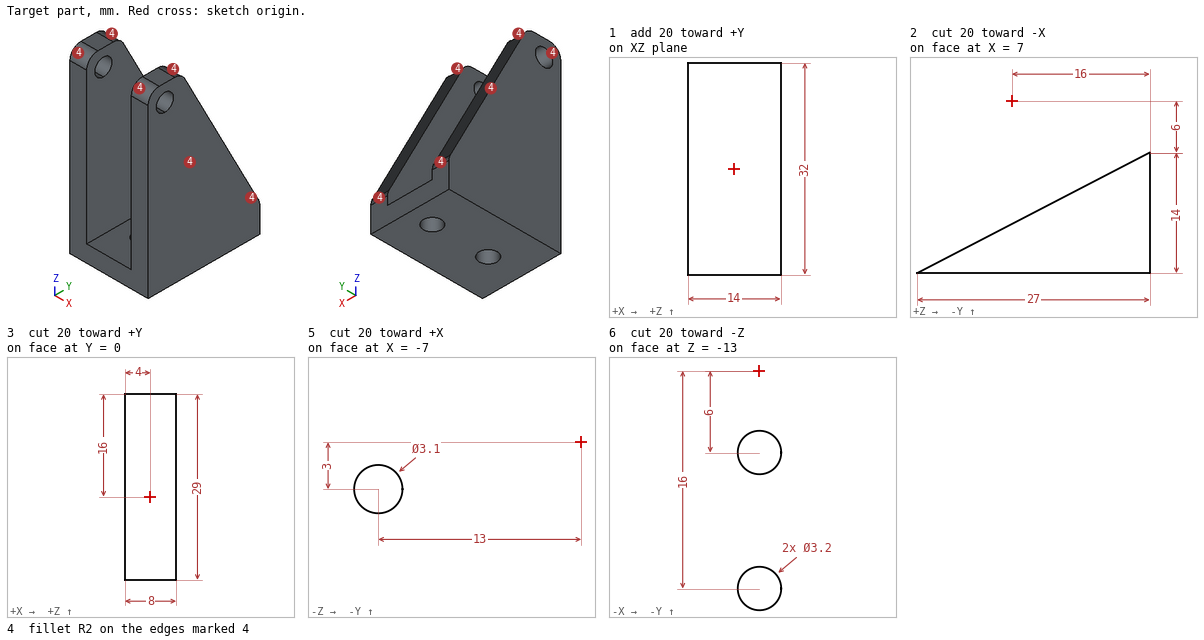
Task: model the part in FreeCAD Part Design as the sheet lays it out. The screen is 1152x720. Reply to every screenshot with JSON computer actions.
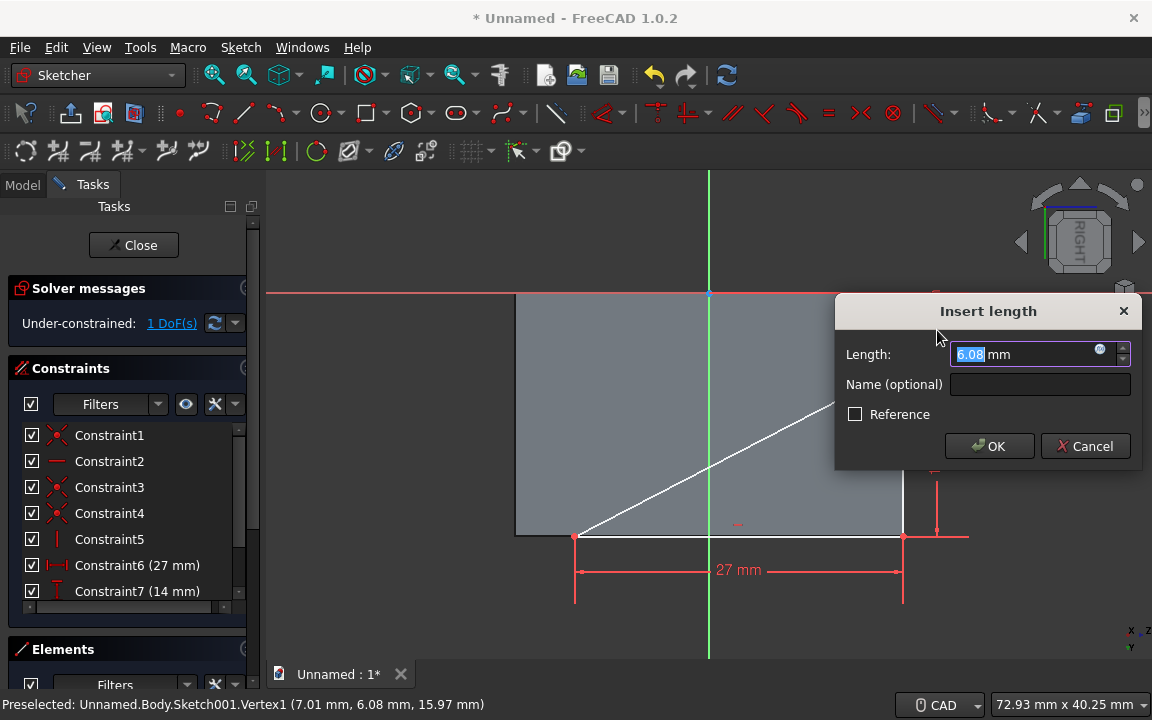
{"action": "type", "text": "6"}
{"action": "key", "text": "Return"}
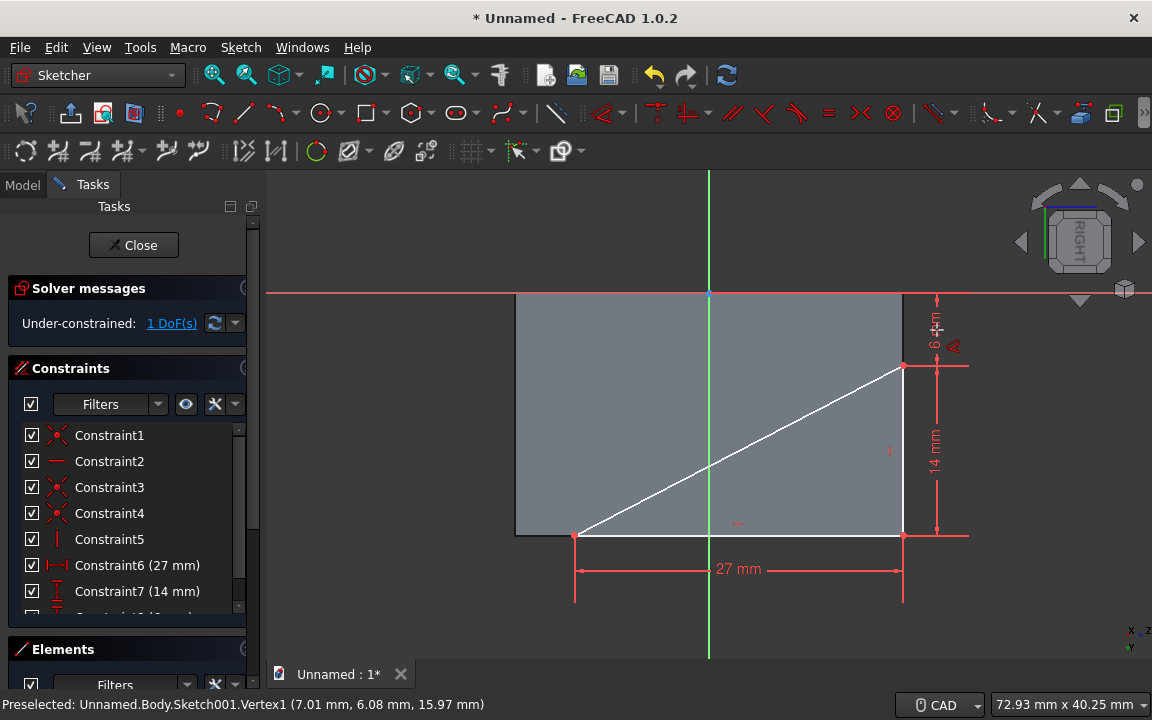
{"action": "left_click", "coordinate": [903, 366]}
{"action": "left_click", "coordinate": [806, 259]}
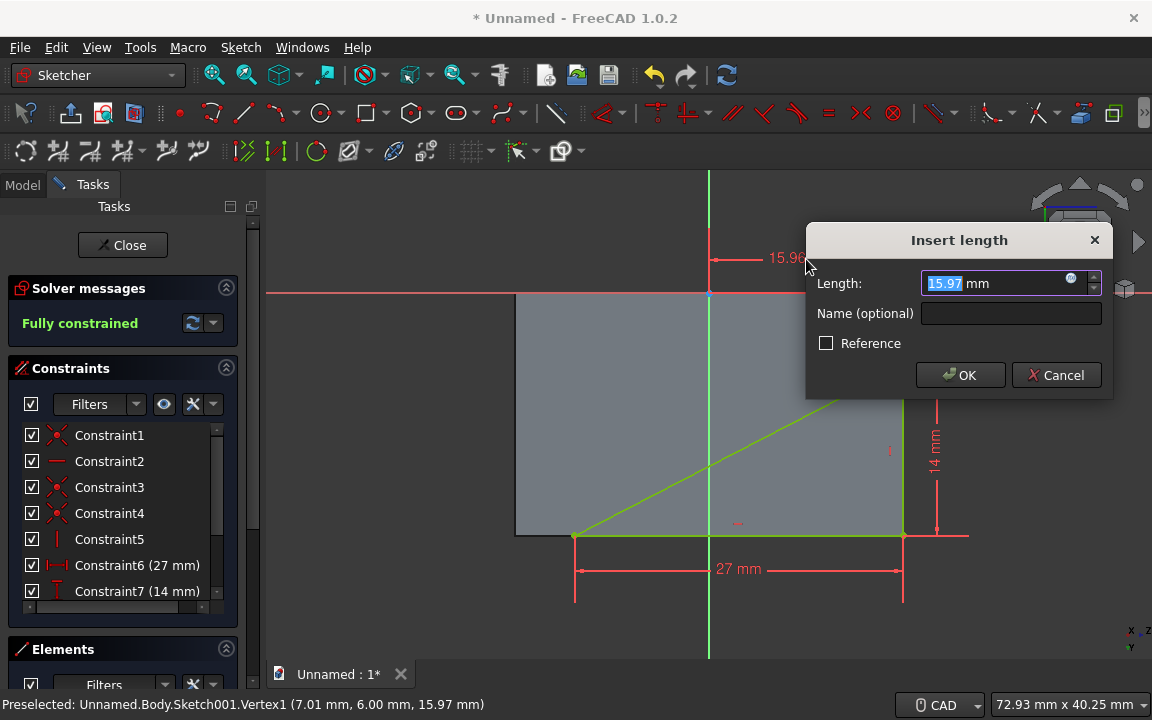
{"action": "type", "text": "16"}
{"action": "key", "text": "Return"}
{"action": "key", "text": "Escape"}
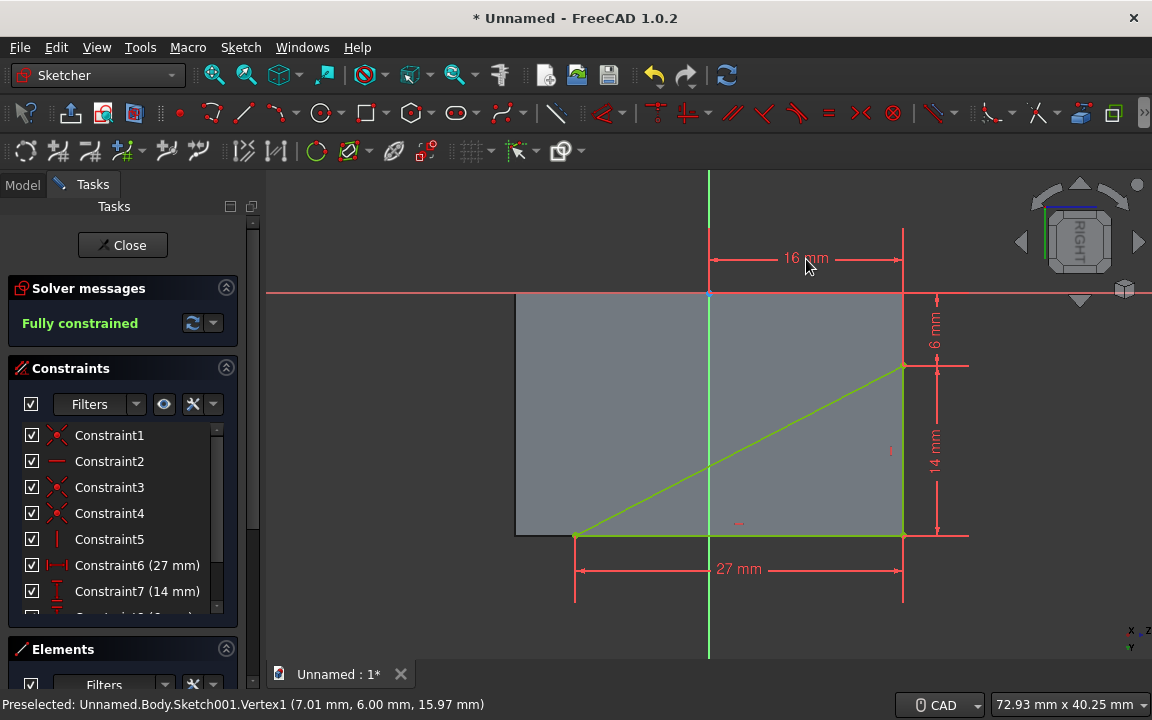
{"action": "left_click", "coordinate": [123, 245]}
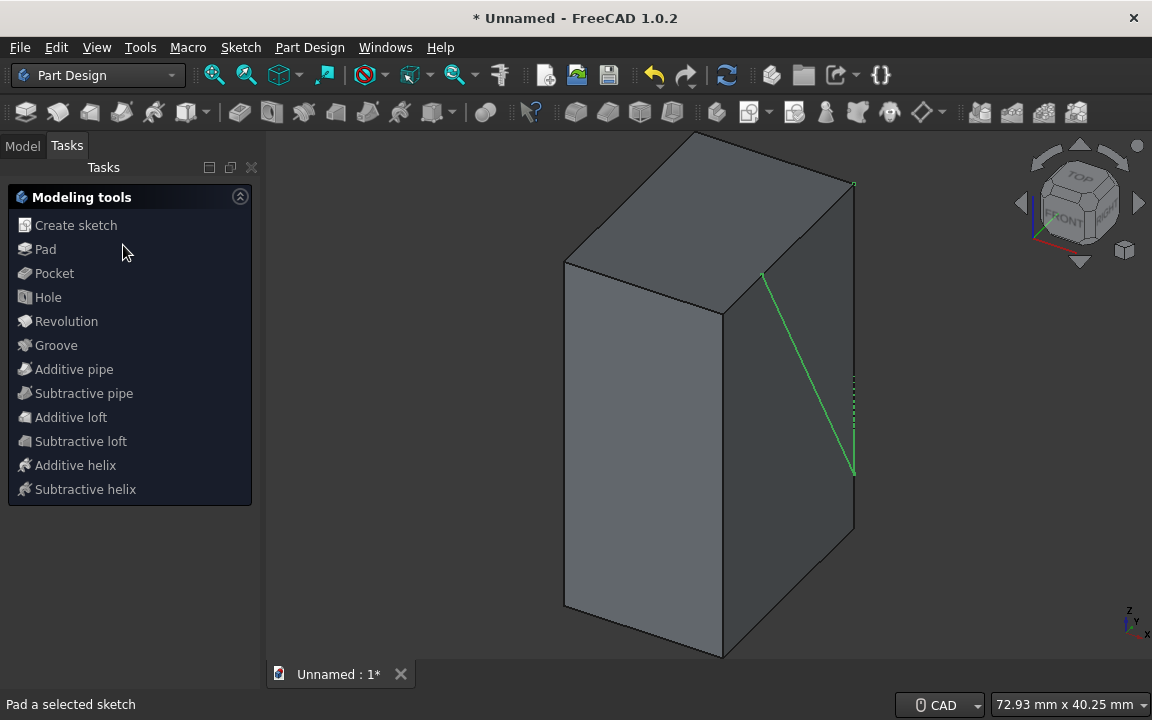
{"action": "left_click", "coordinate": [240, 112]}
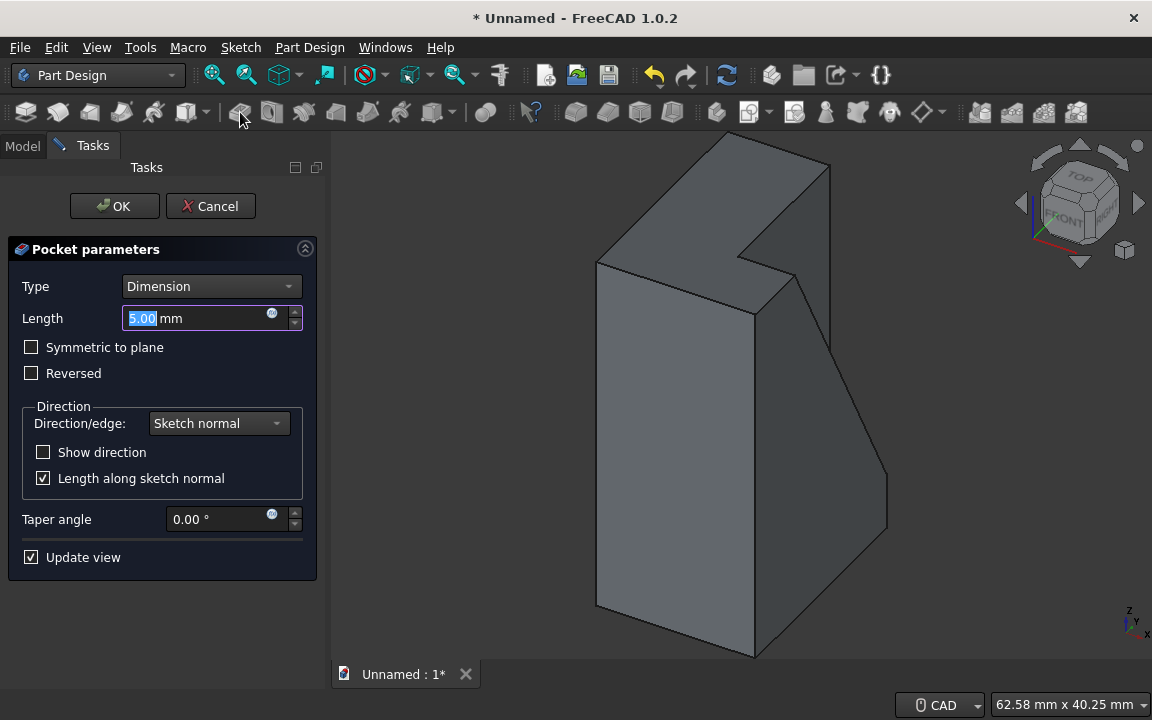
{"action": "type", "text": "20"}
{"action": "key", "text": "Tab"}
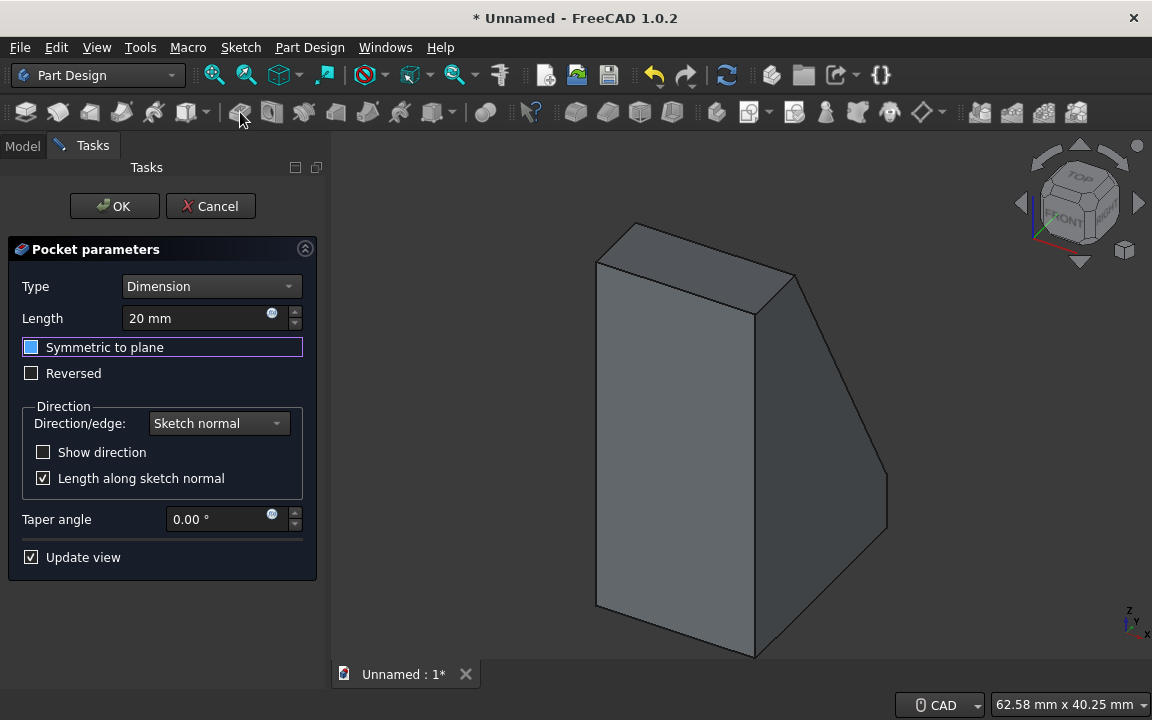
{"action": "left_click", "coordinate": [115, 206]}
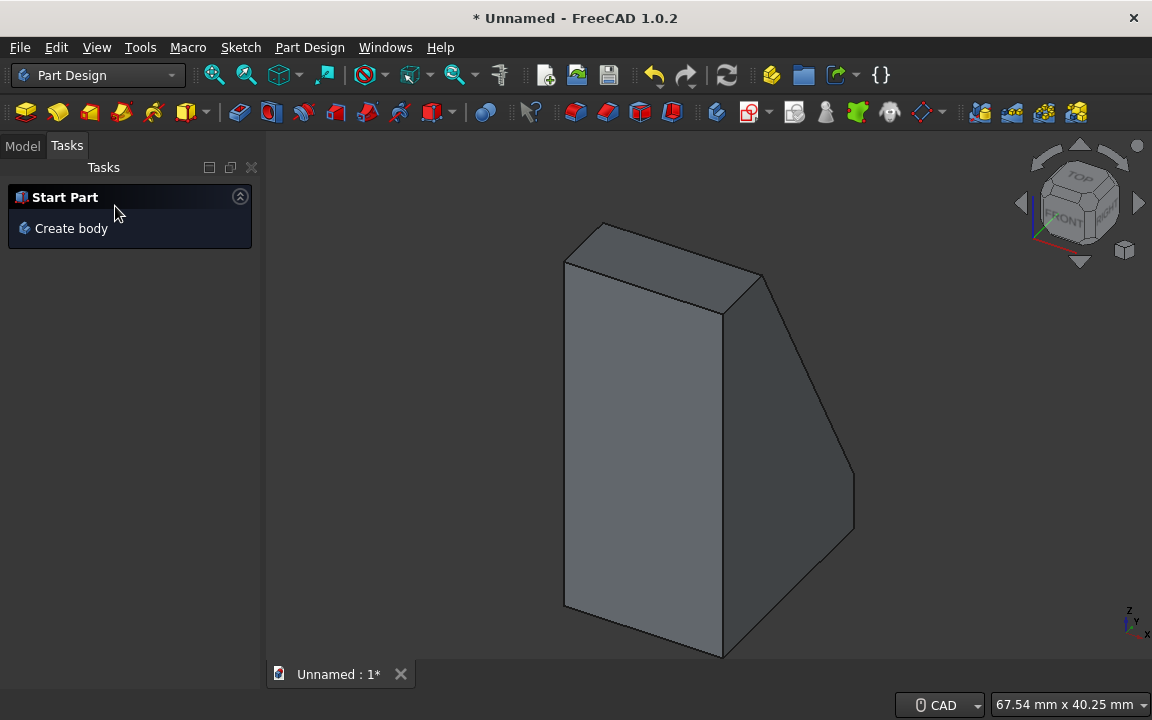
{"action": "left_click", "coordinate": [643, 410]}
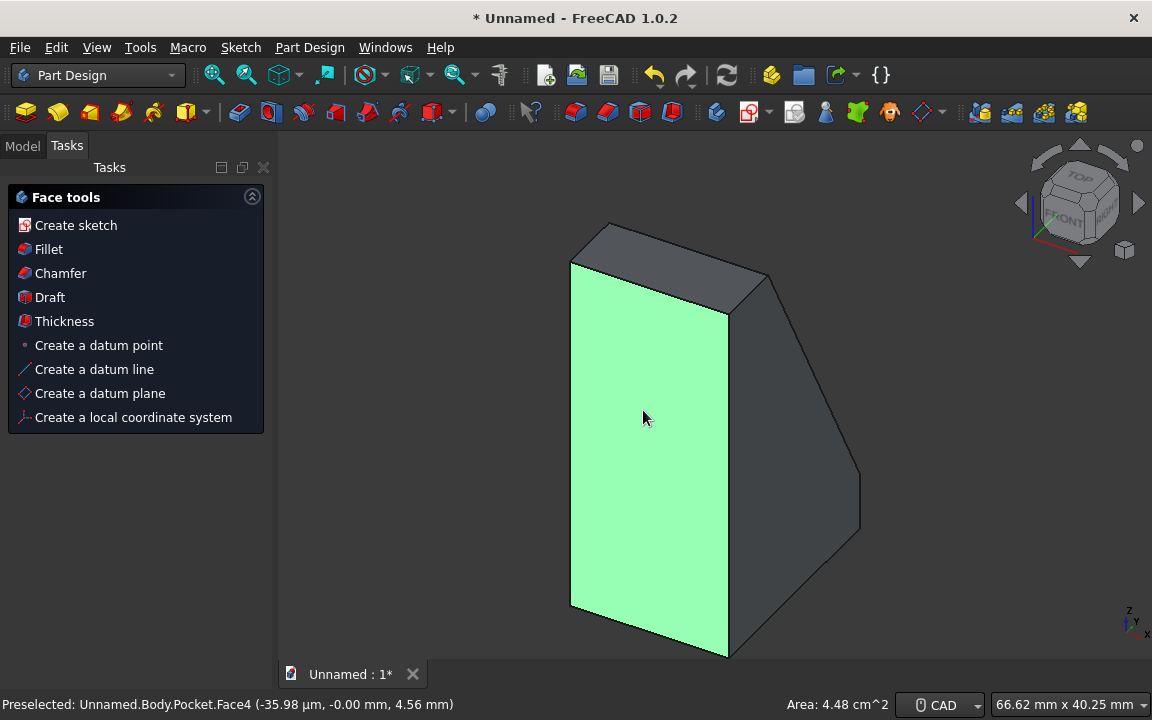
{"action": "left_click", "coordinate": [750, 112]}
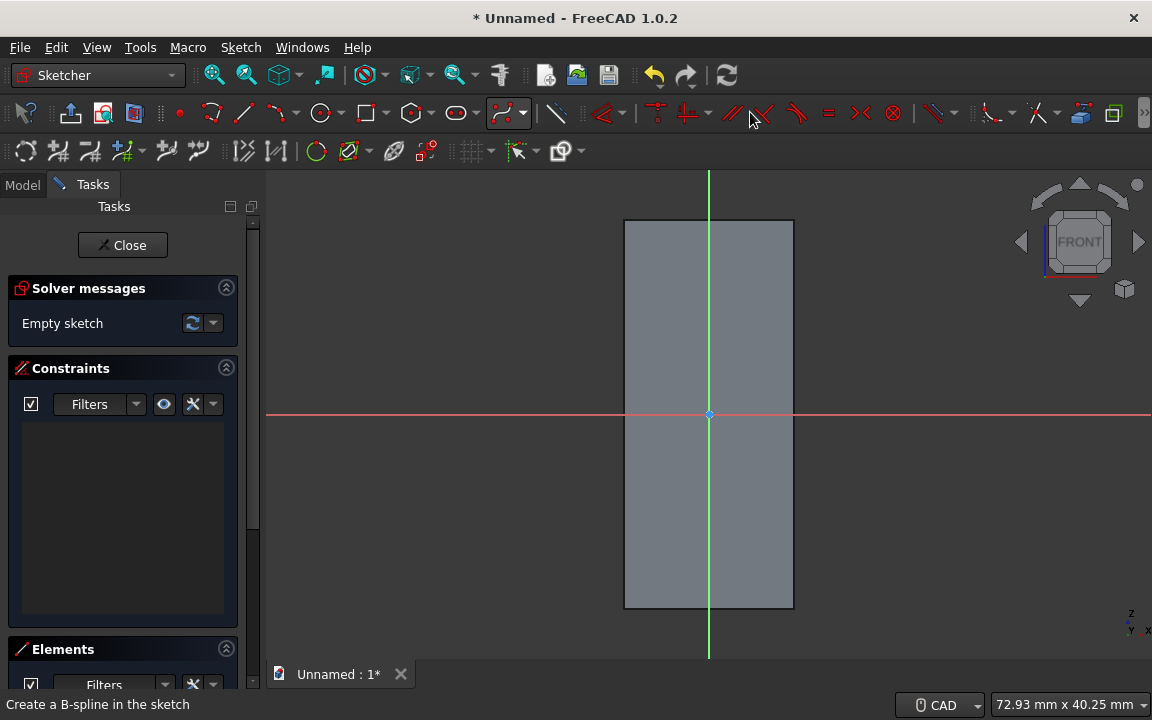
{"action": "scroll", "coordinate": [331, 497], "scroll_direction": "down", "scroll_amount": 1}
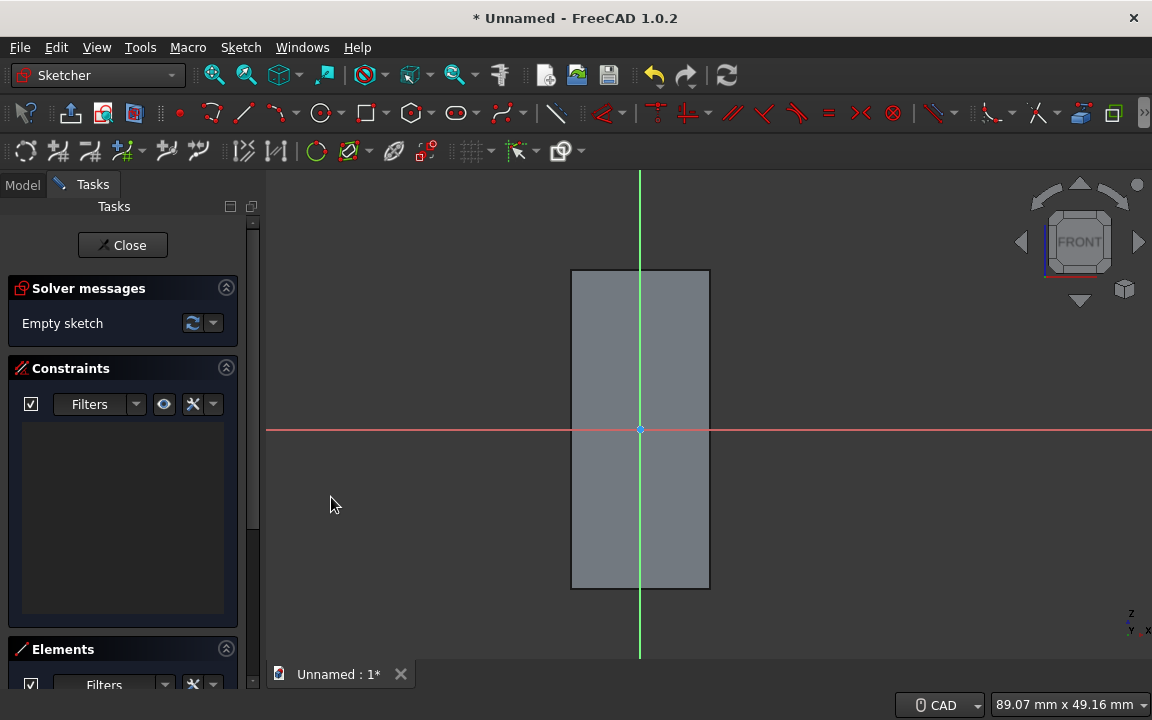
{"action": "key", "text": "g r"}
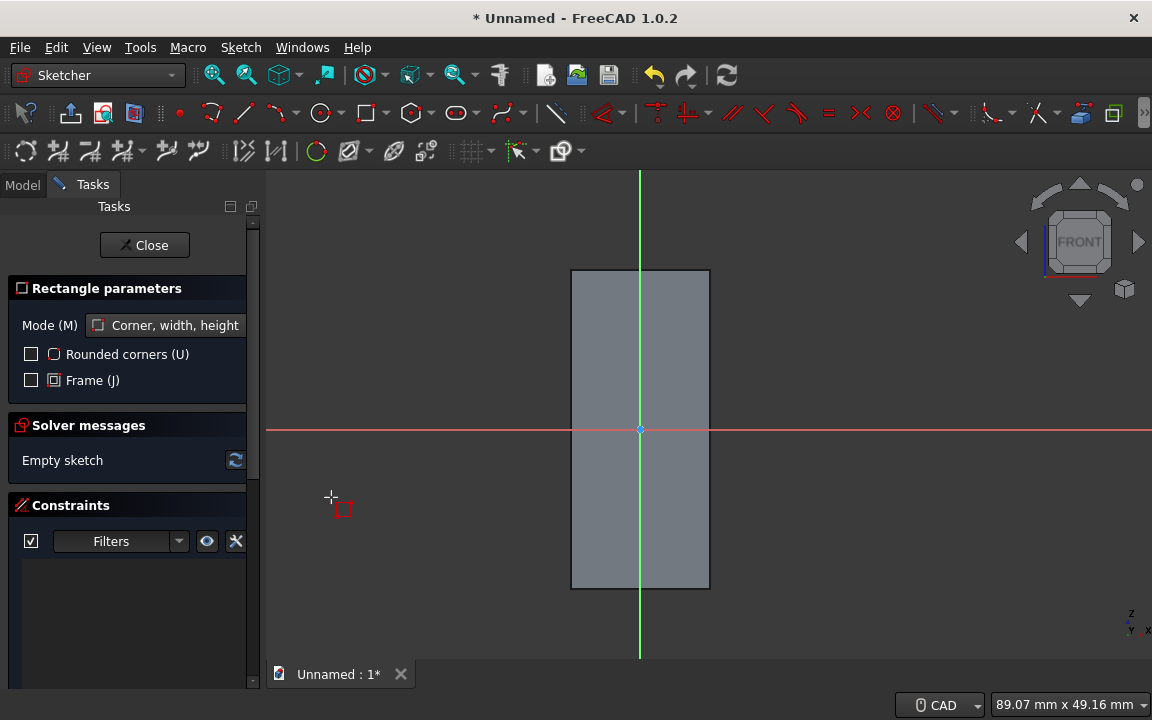
{"action": "left_click", "coordinate": [601, 270]}
{"action": "mouse_move", "coordinate": [680, 559]}